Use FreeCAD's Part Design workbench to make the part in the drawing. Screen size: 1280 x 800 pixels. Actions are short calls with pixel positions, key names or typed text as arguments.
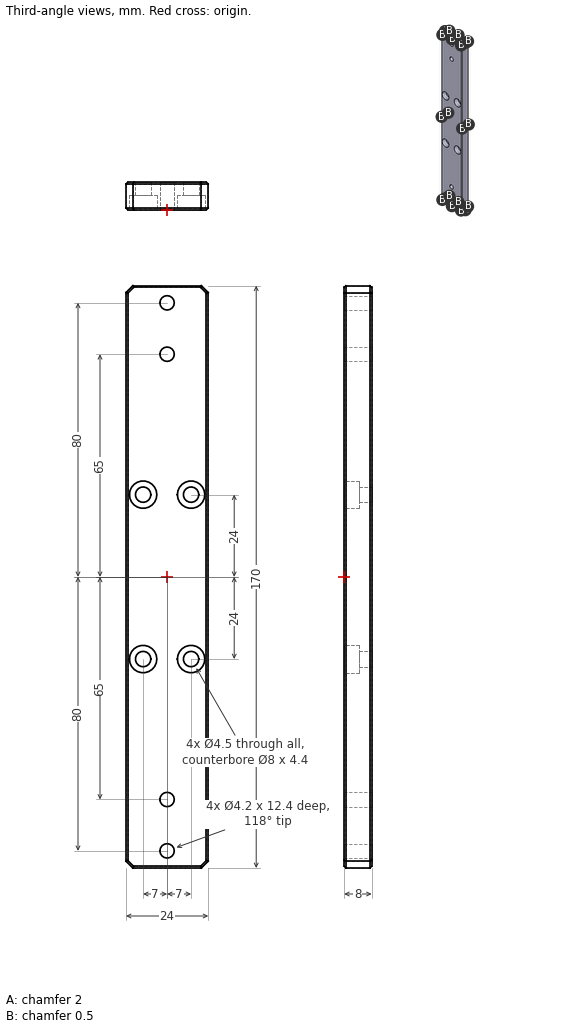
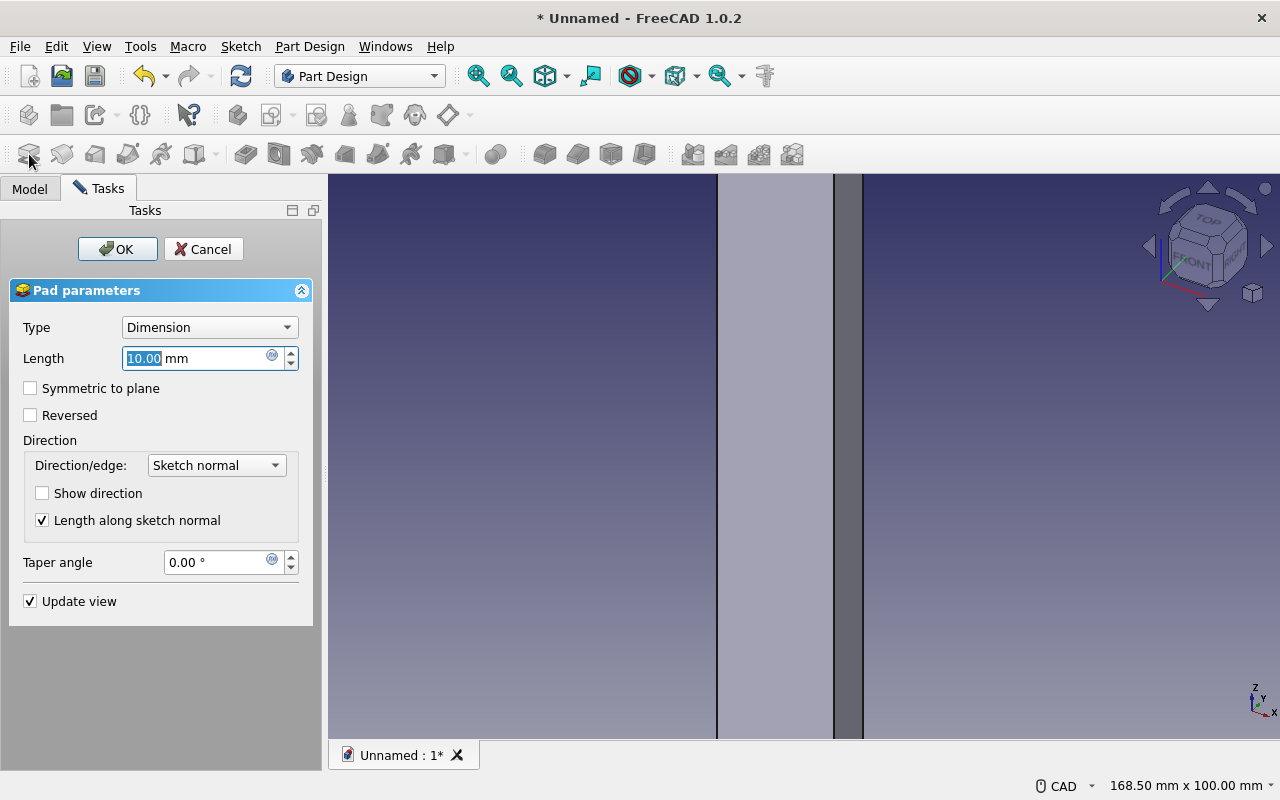
text(8)
key(Tab)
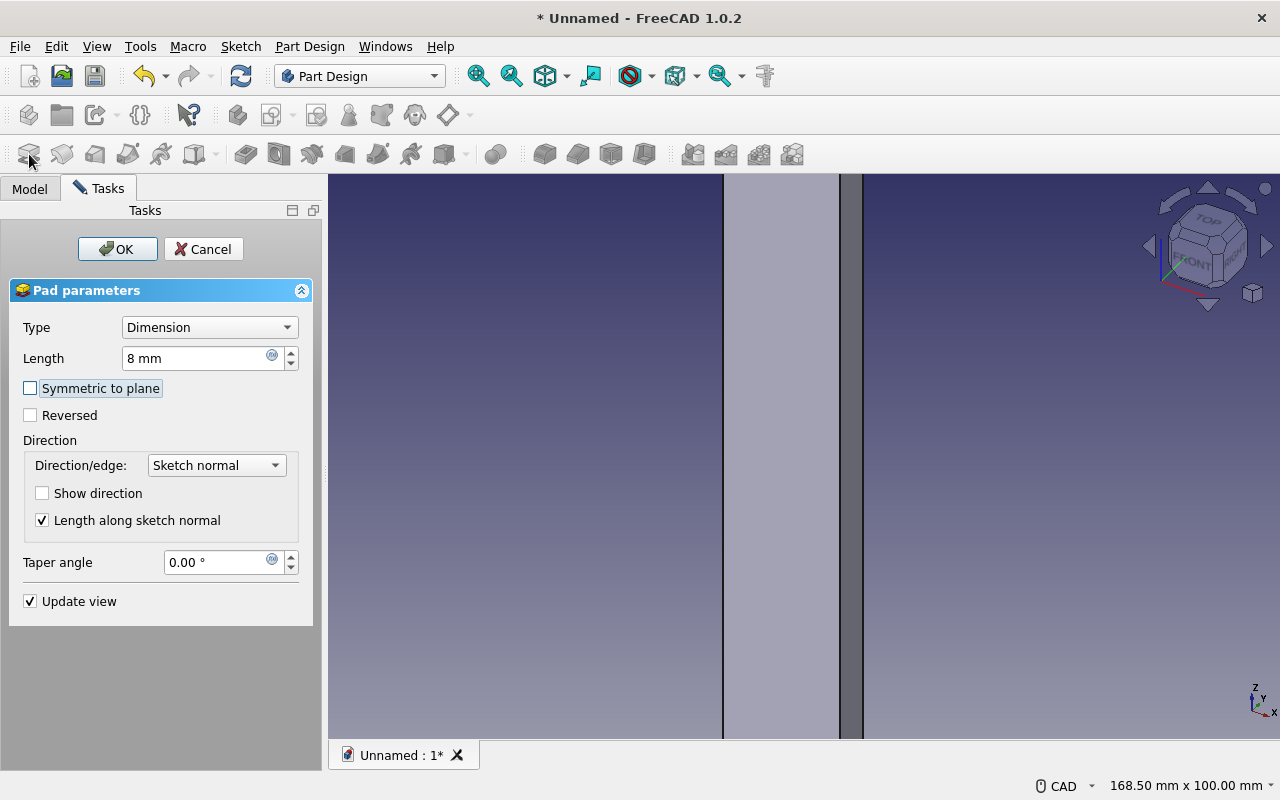
click(31, 415)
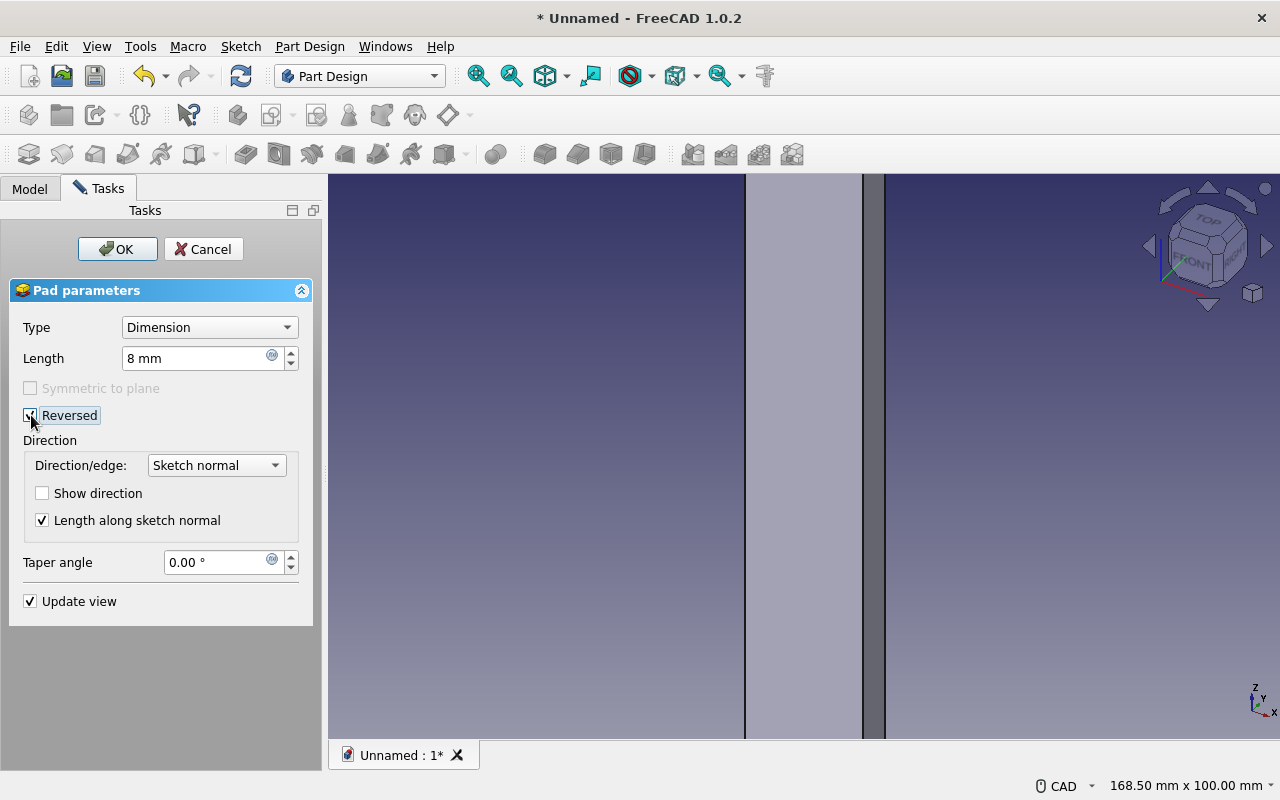
click(118, 249)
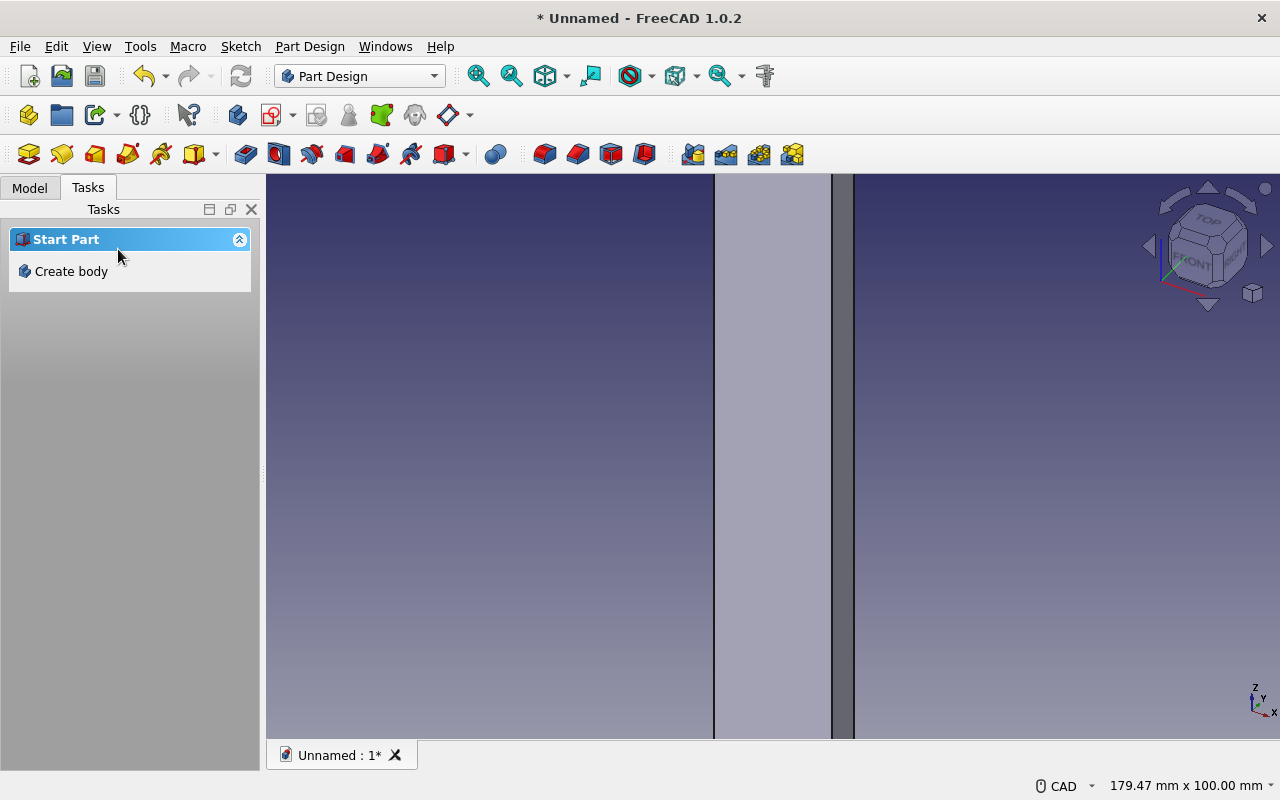
click(479, 76)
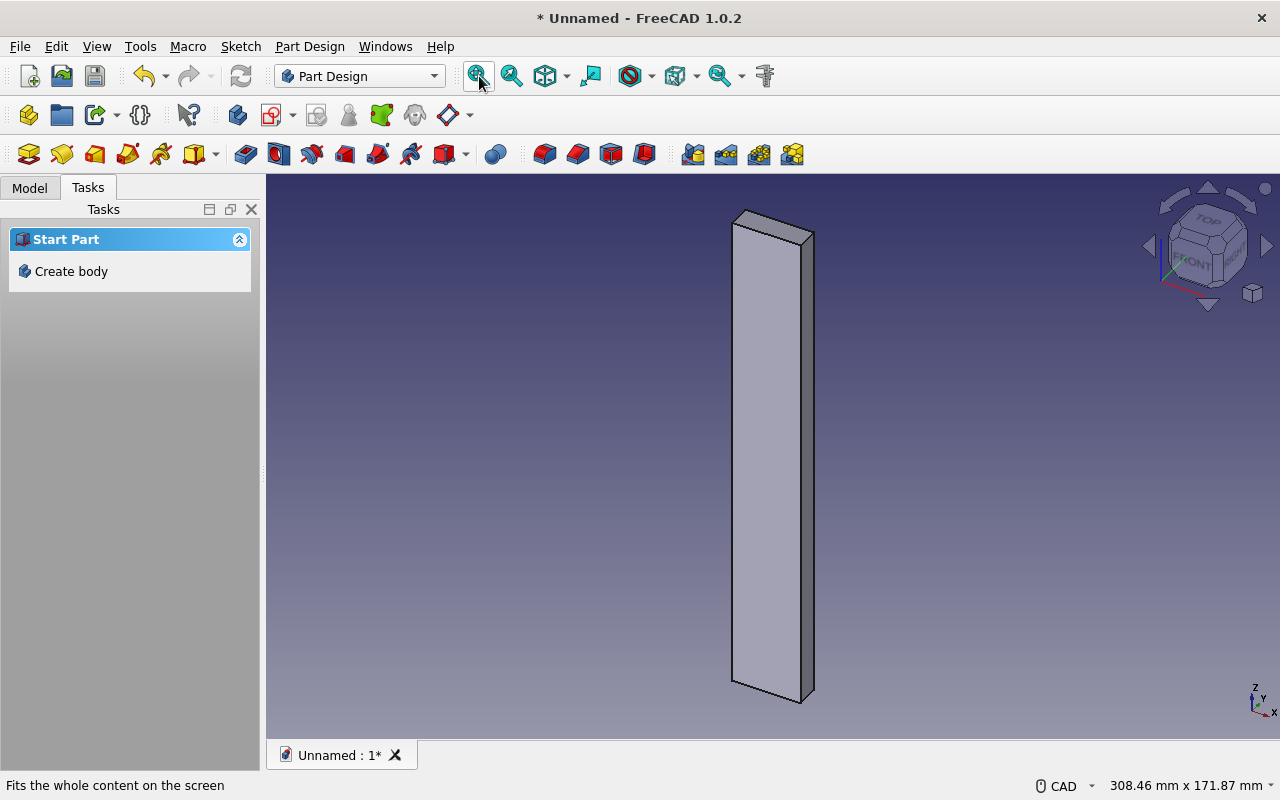
click(766, 266)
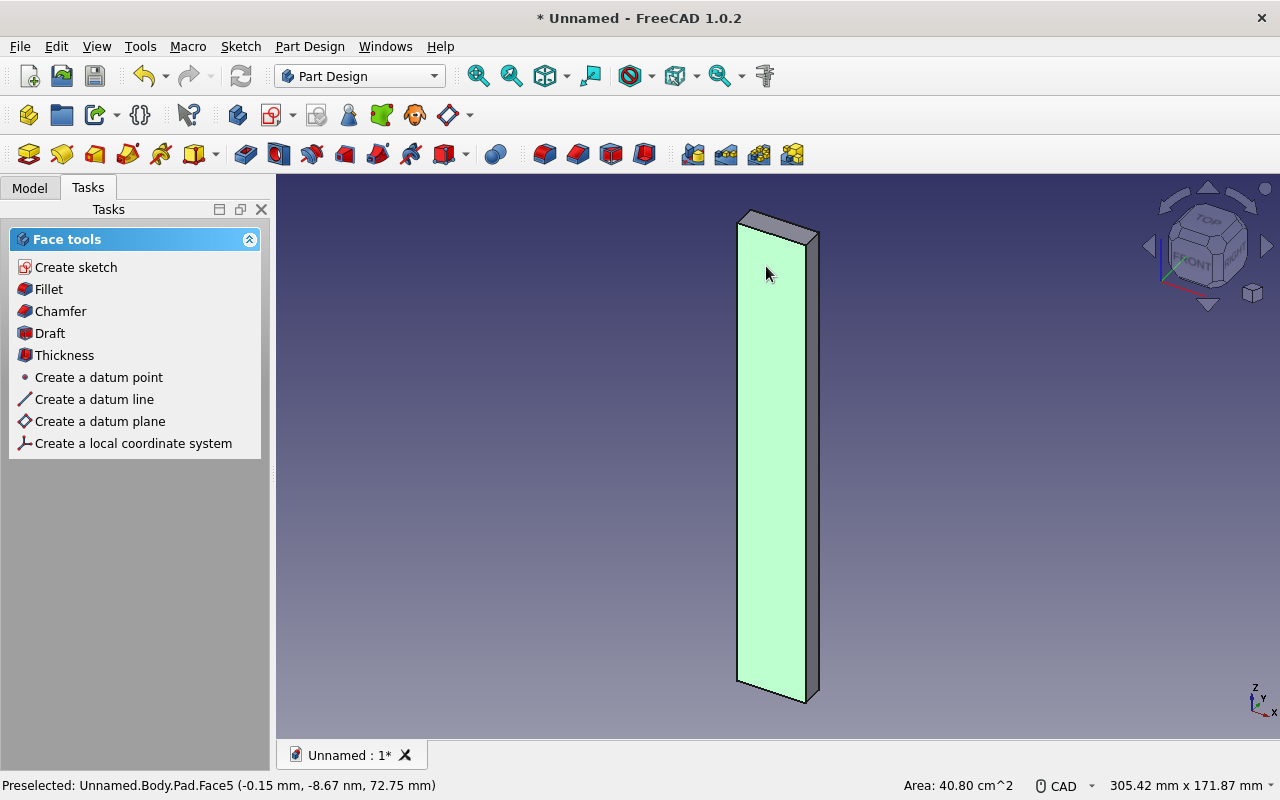
click(270, 116)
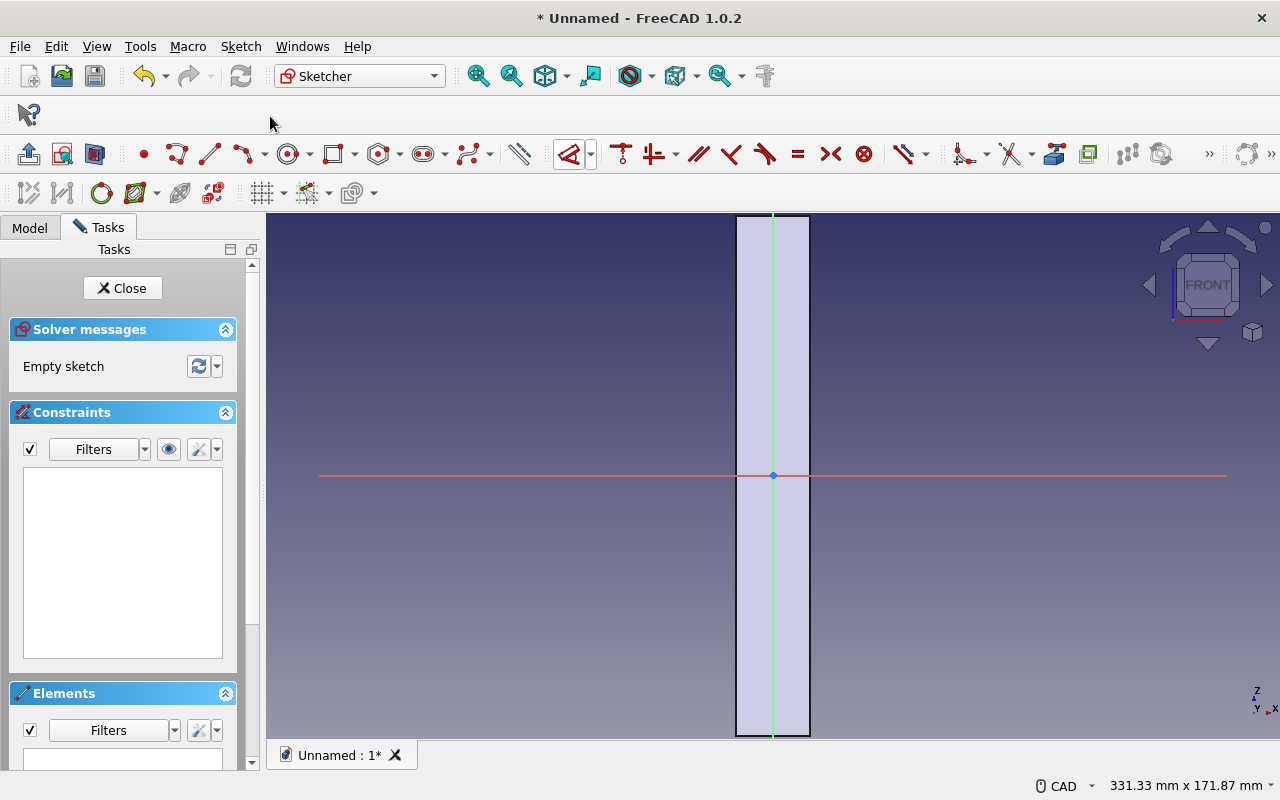
scroll(829, 476, up, 4)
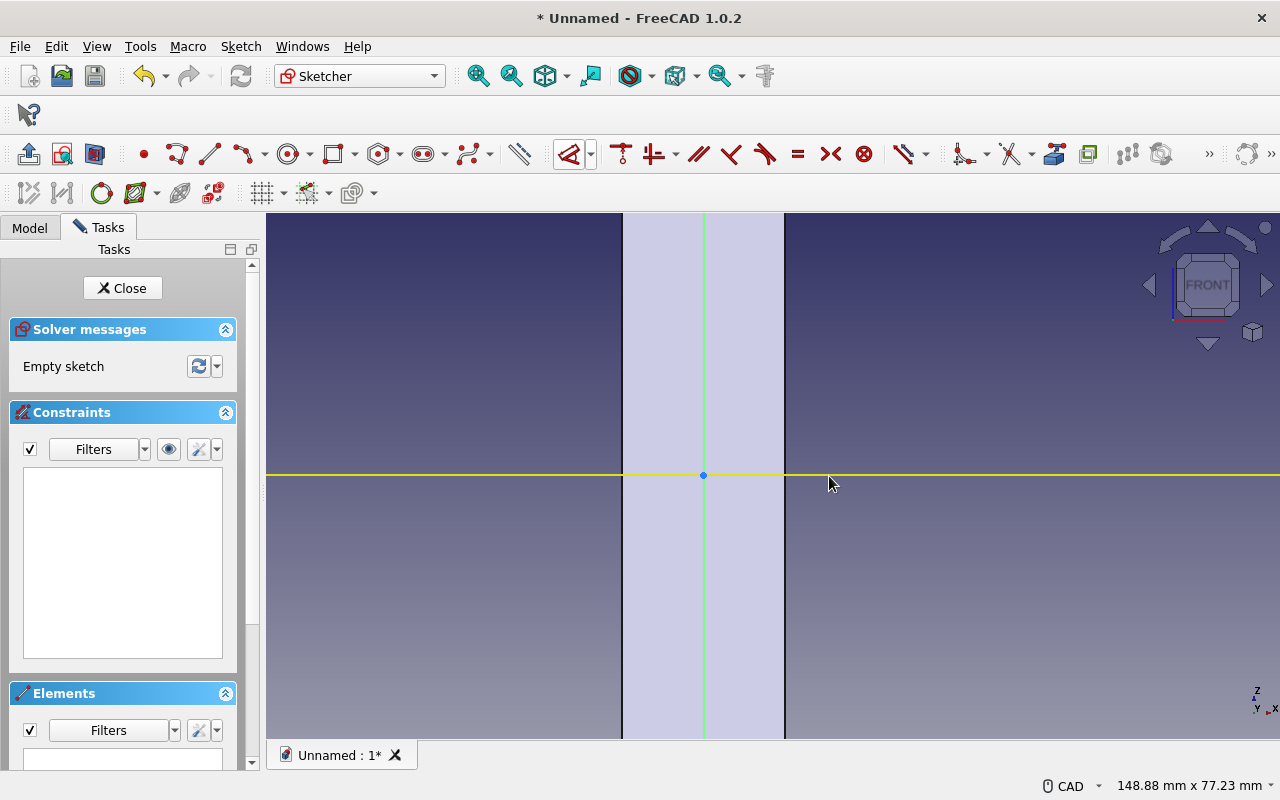
click(288, 154)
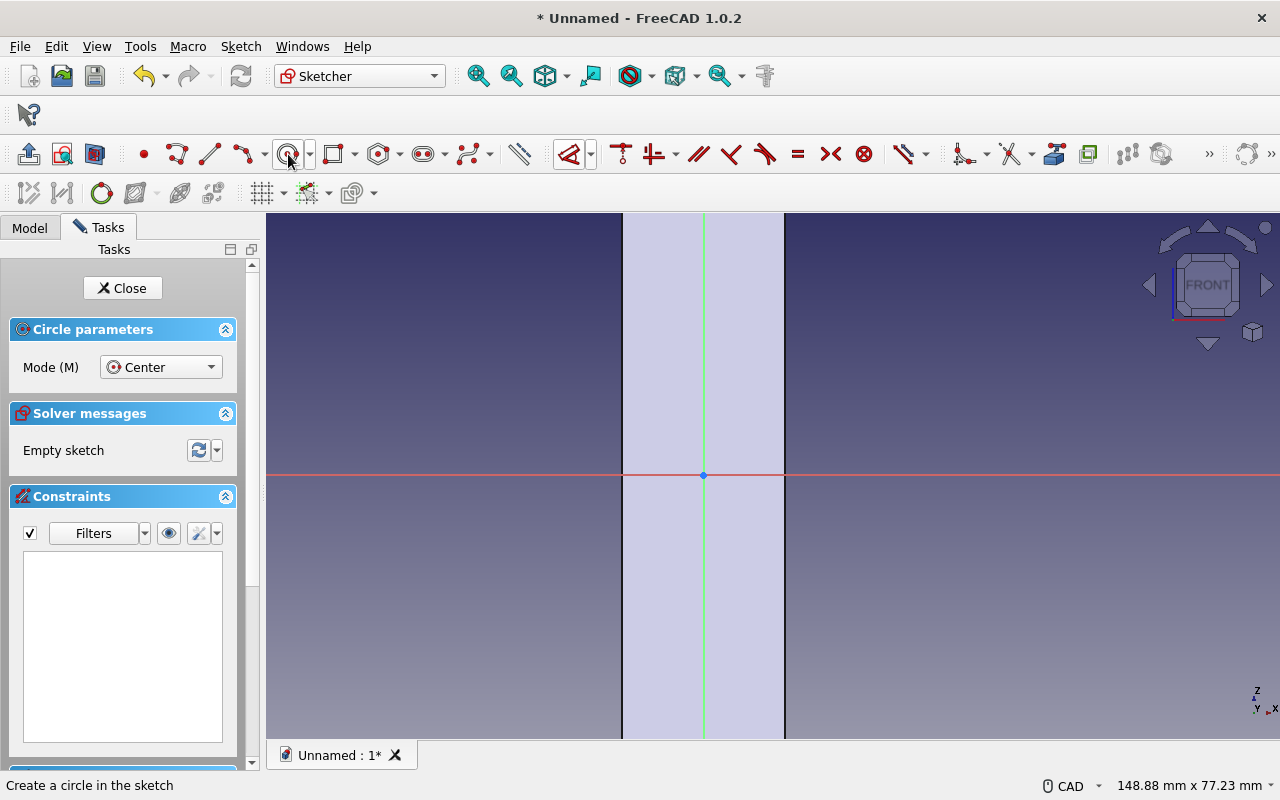
scroll(751, 639, up, 2)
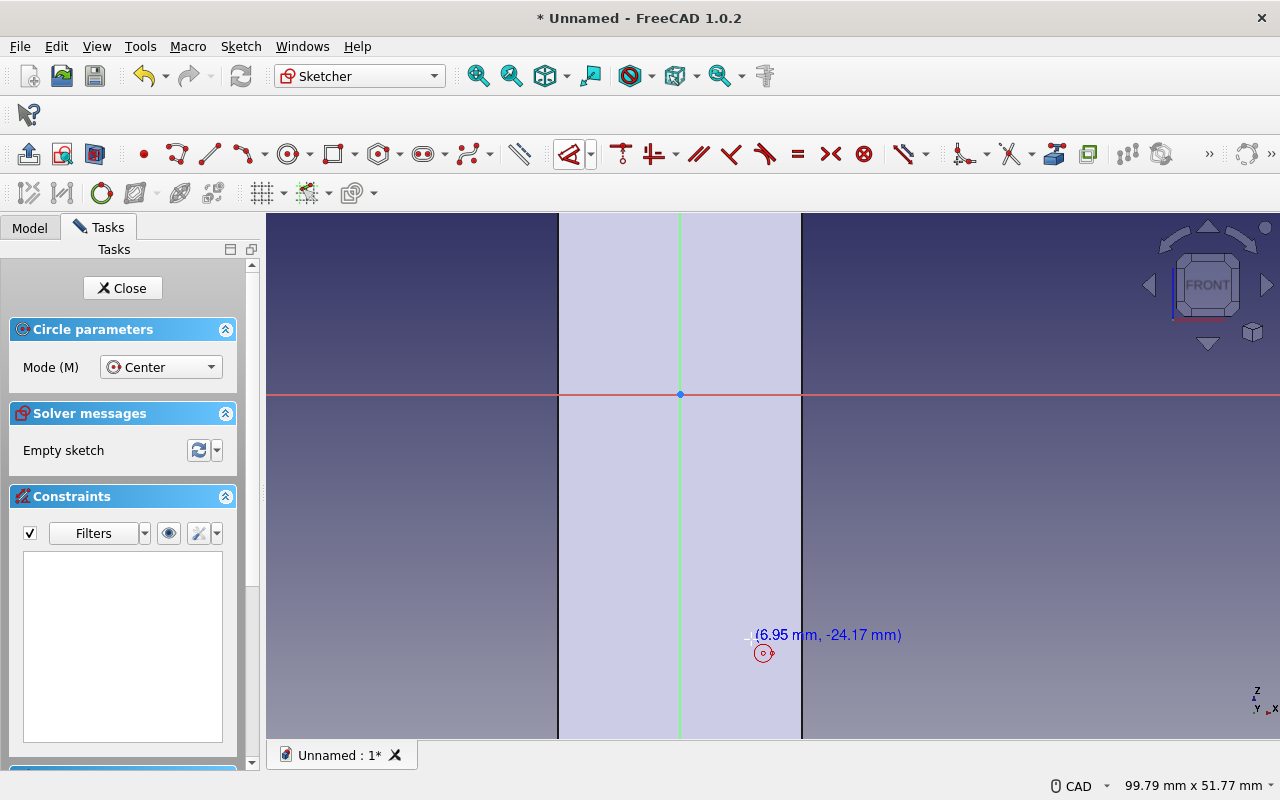
click(751, 638)
move(767, 622)